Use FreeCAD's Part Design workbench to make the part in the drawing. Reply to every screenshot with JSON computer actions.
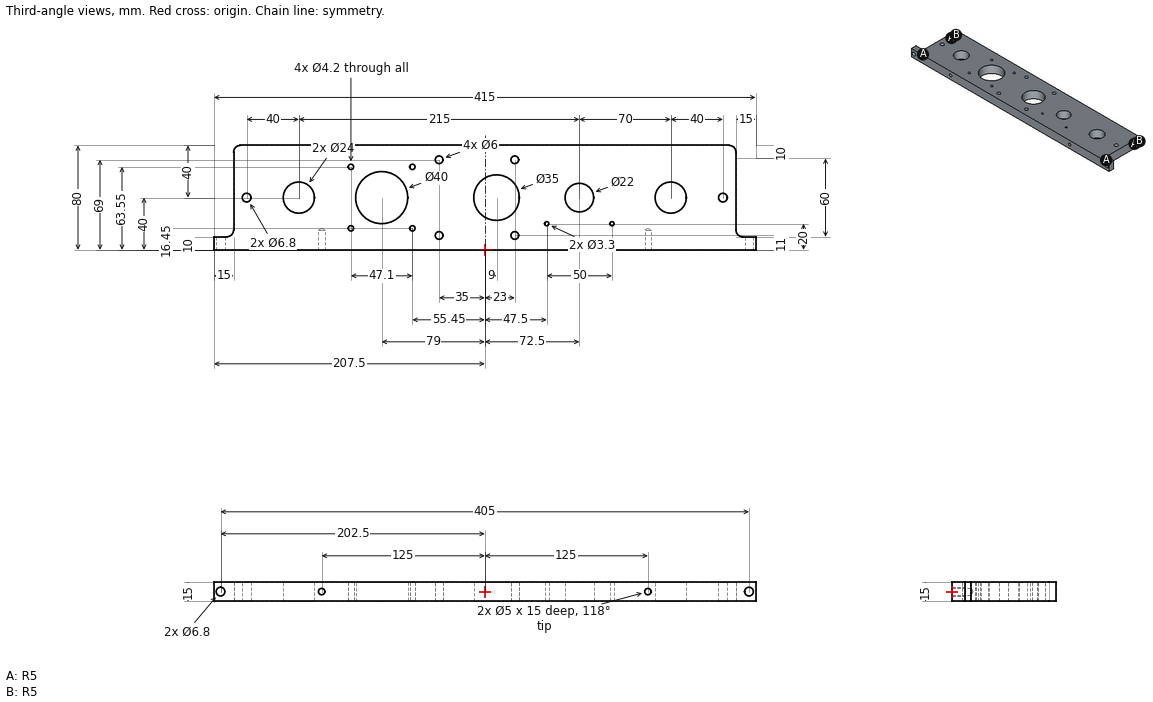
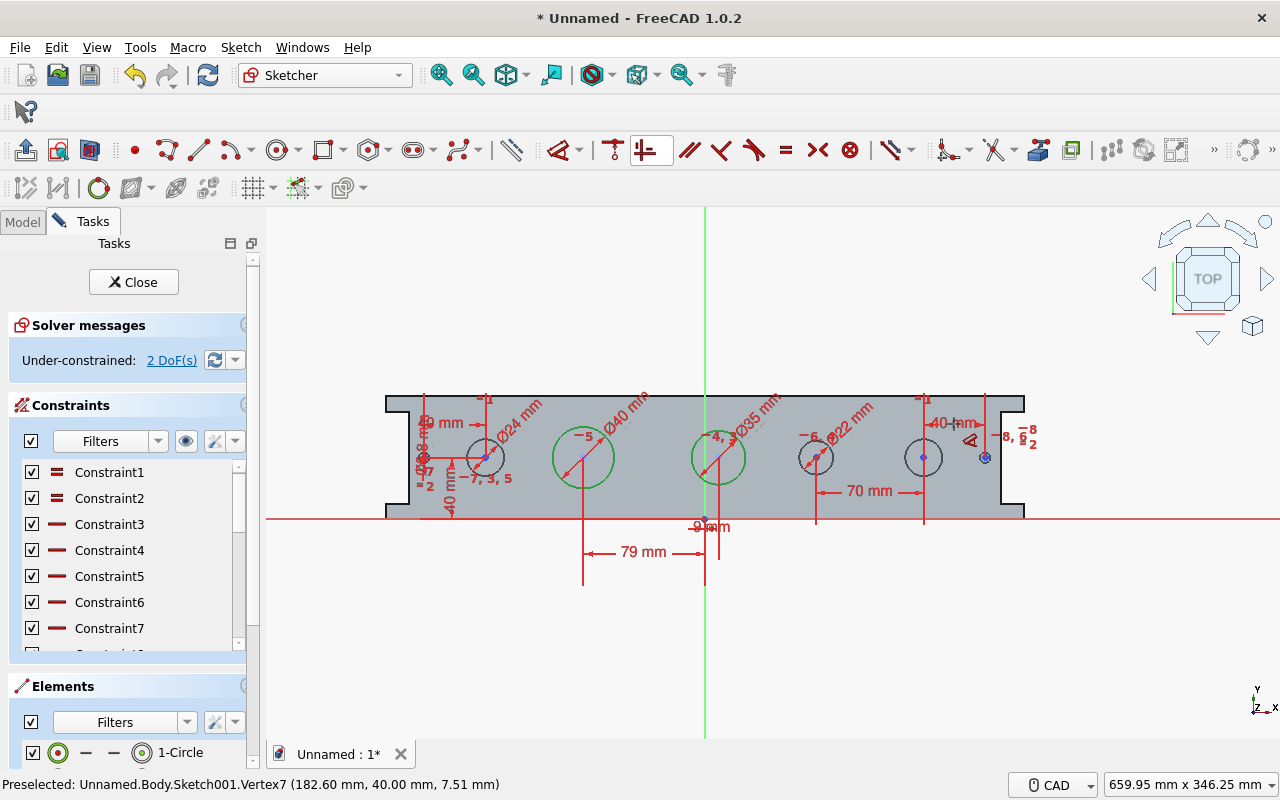
{"action": "left_click", "coordinate": [816, 458]}
{"action": "left_click", "coordinate": [760, 553]}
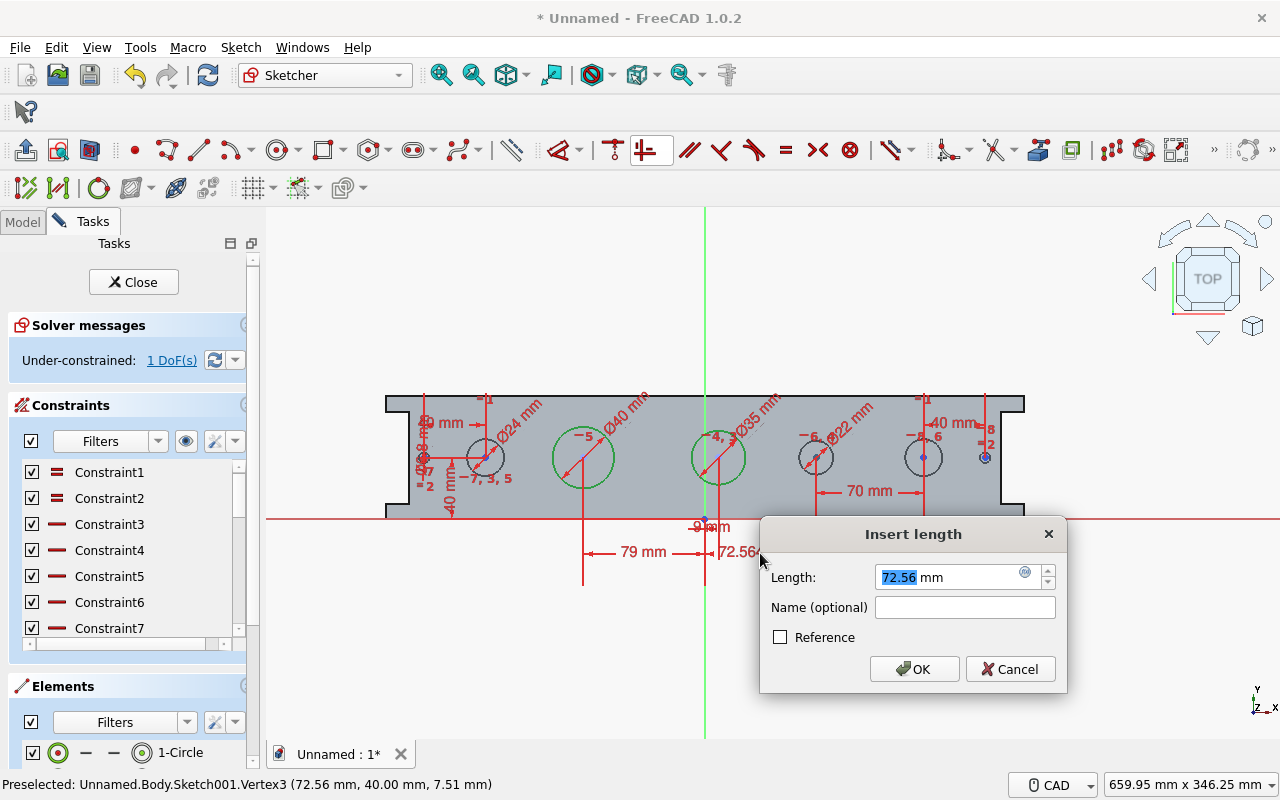
{"action": "type", "text": "72.5"}
{"action": "key", "text": "Return"}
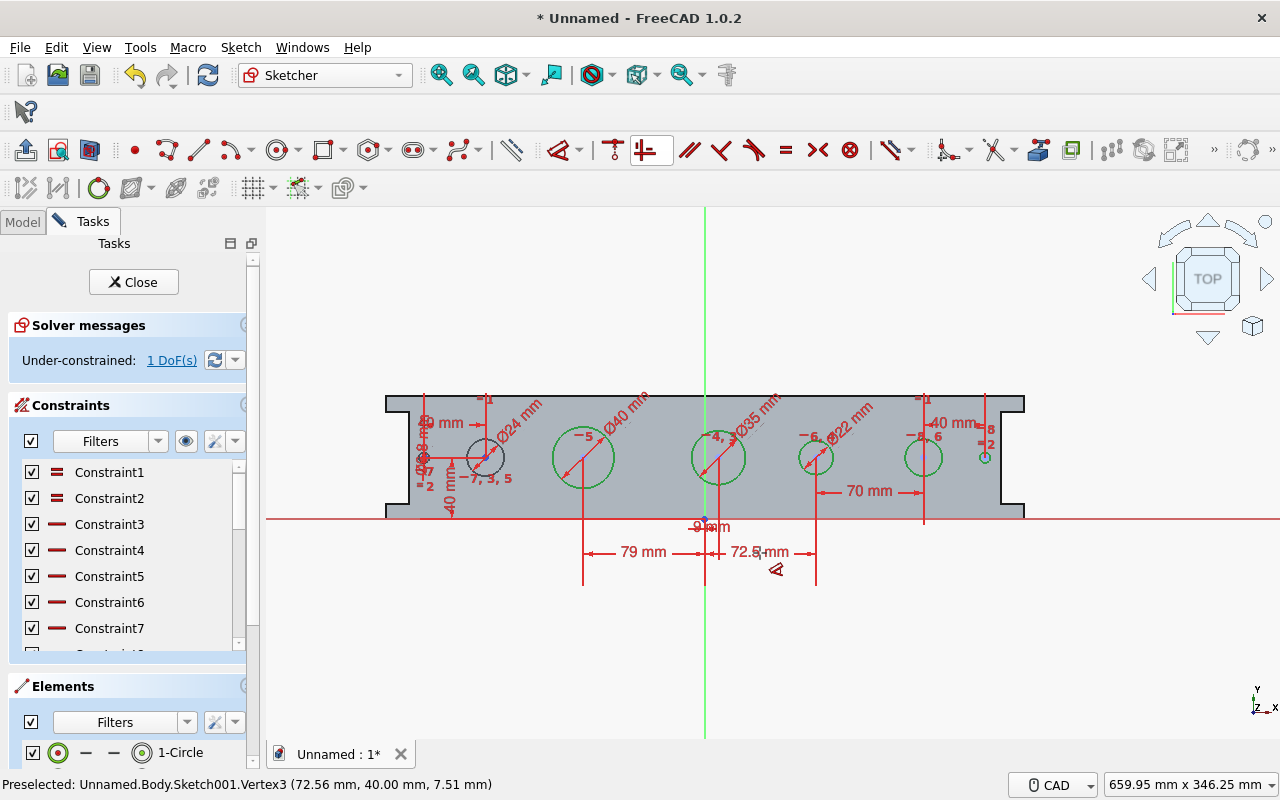
{"action": "left_click", "coordinate": [486, 458]}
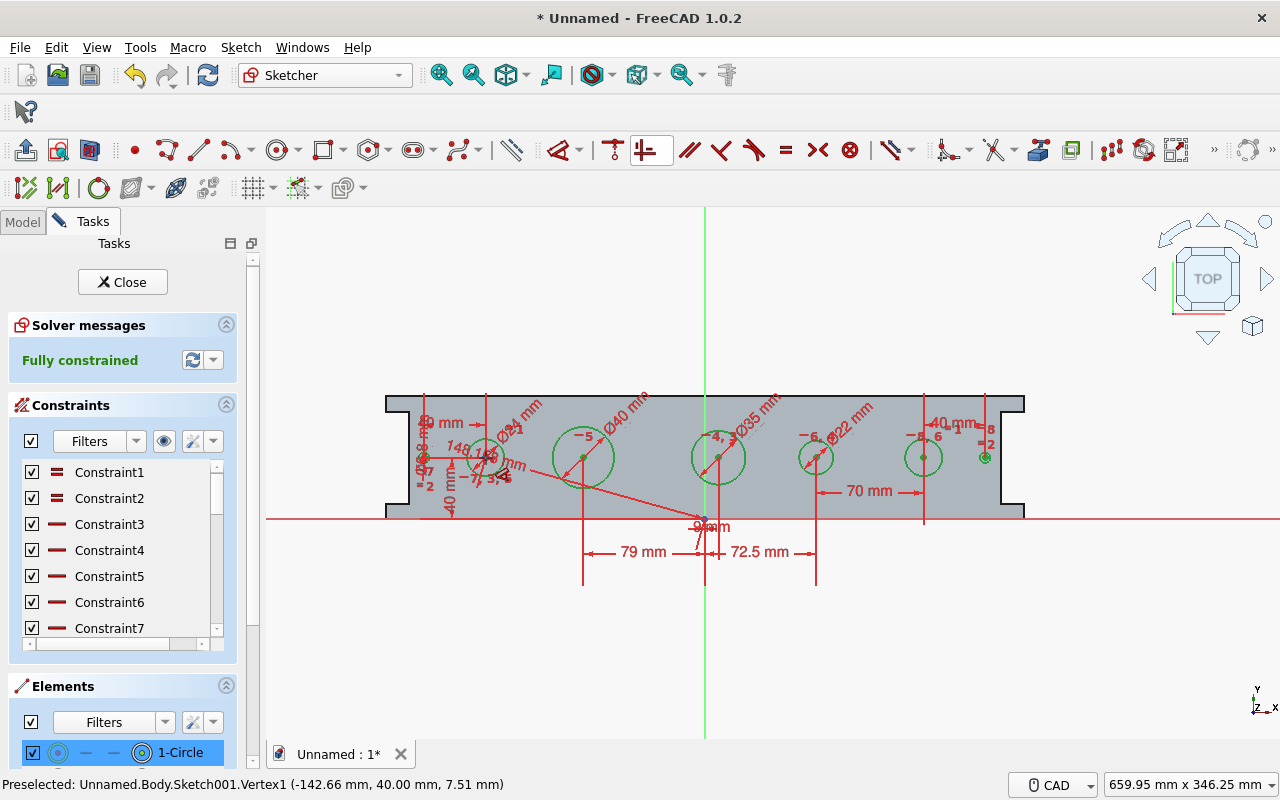
{"action": "left_click", "coordinate": [816, 458]}
{"action": "left_click", "coordinate": [651, 492]}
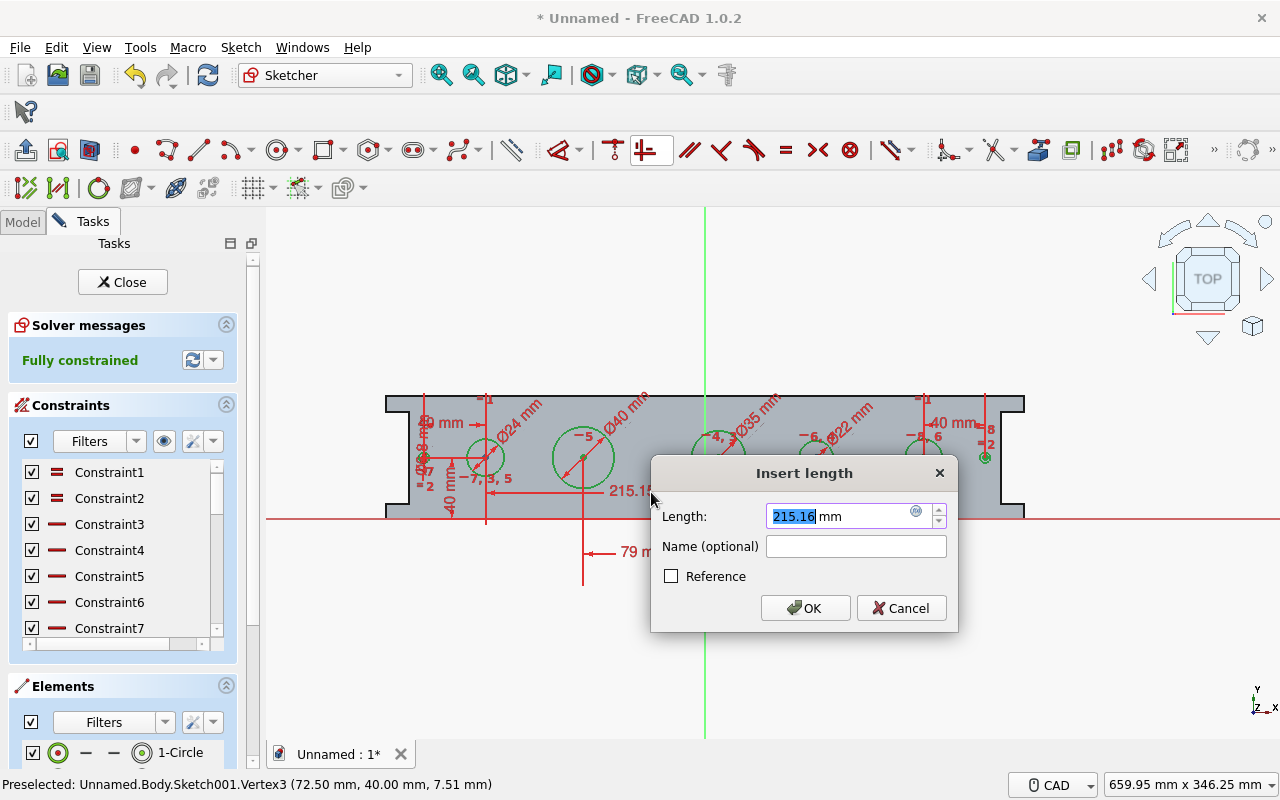
{"action": "type", "text": "215"}
{"action": "key", "text": "Return"}
{"action": "key", "text": "Escape"}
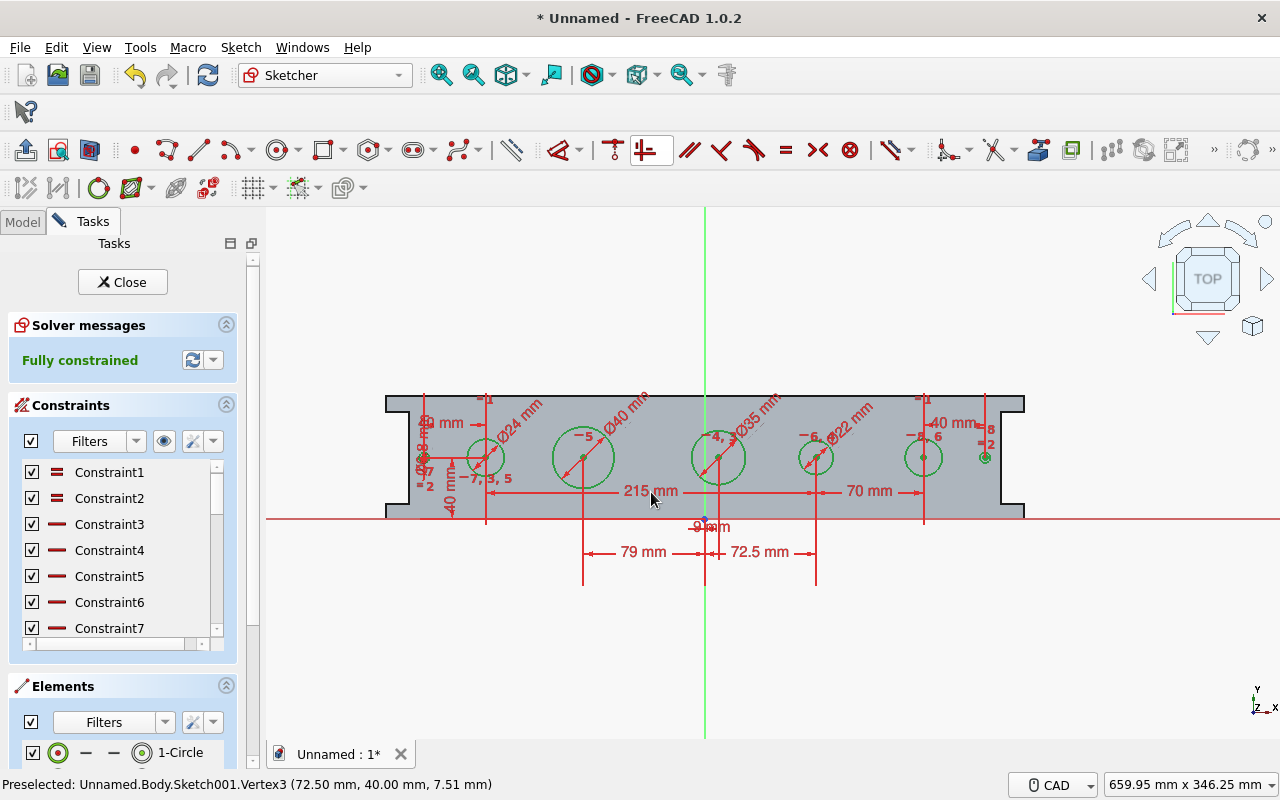
{"action": "left_click", "coordinate": [123, 282]}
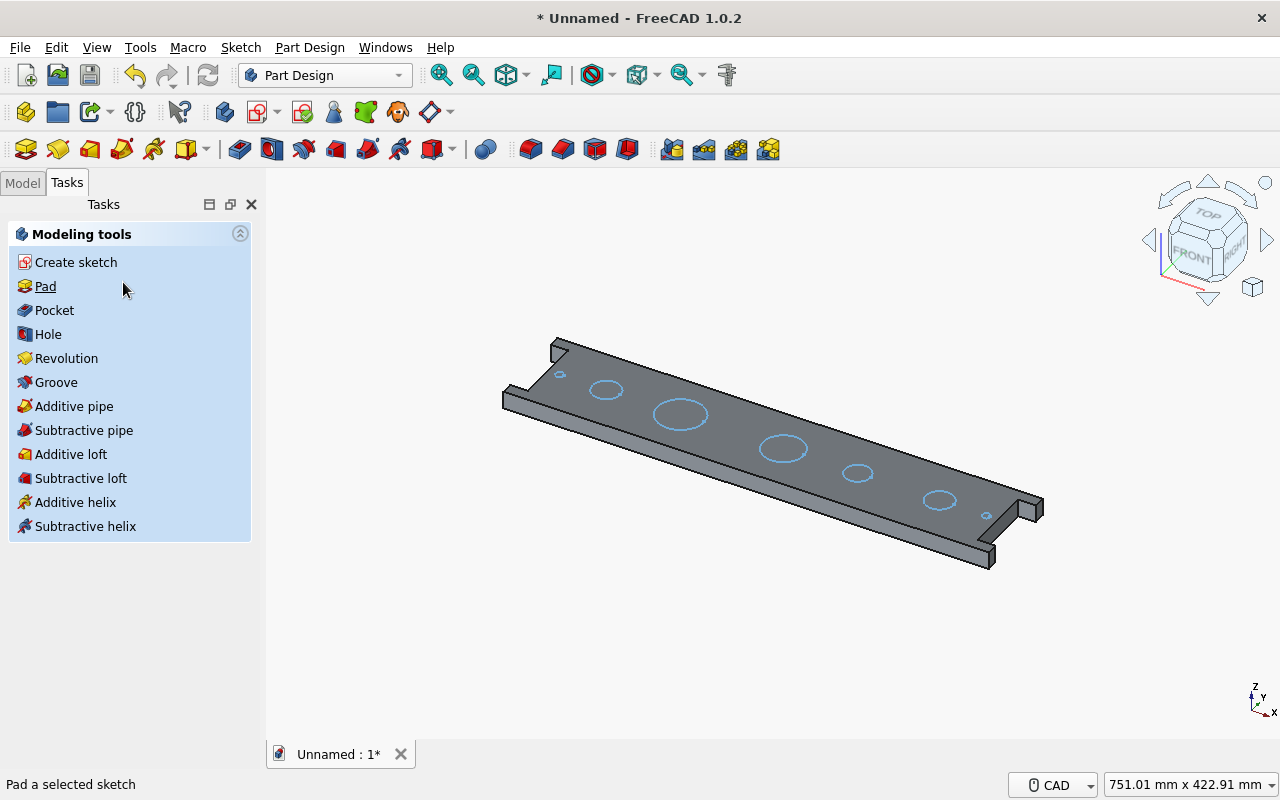
{"action": "left_click", "coordinate": [240, 150]}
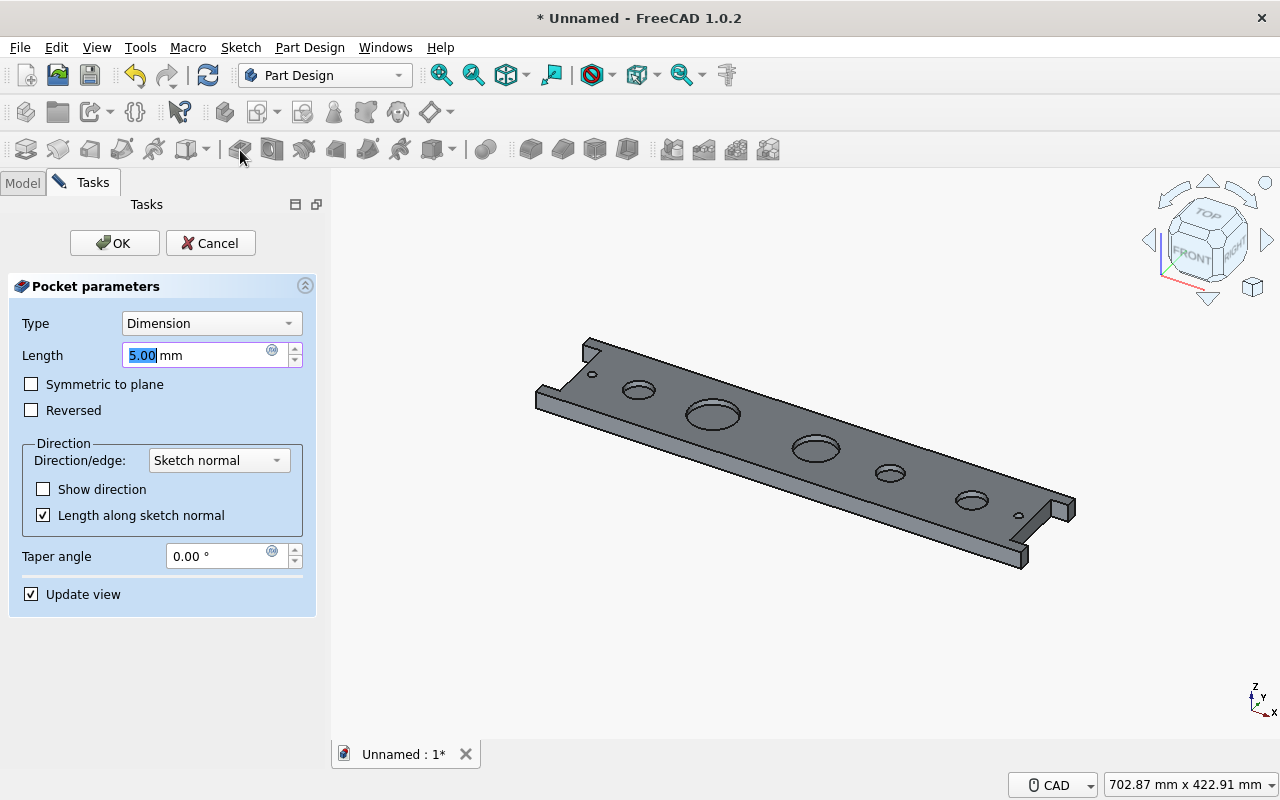
{"action": "type", "text": "15"}
{"action": "key", "text": "Tab"}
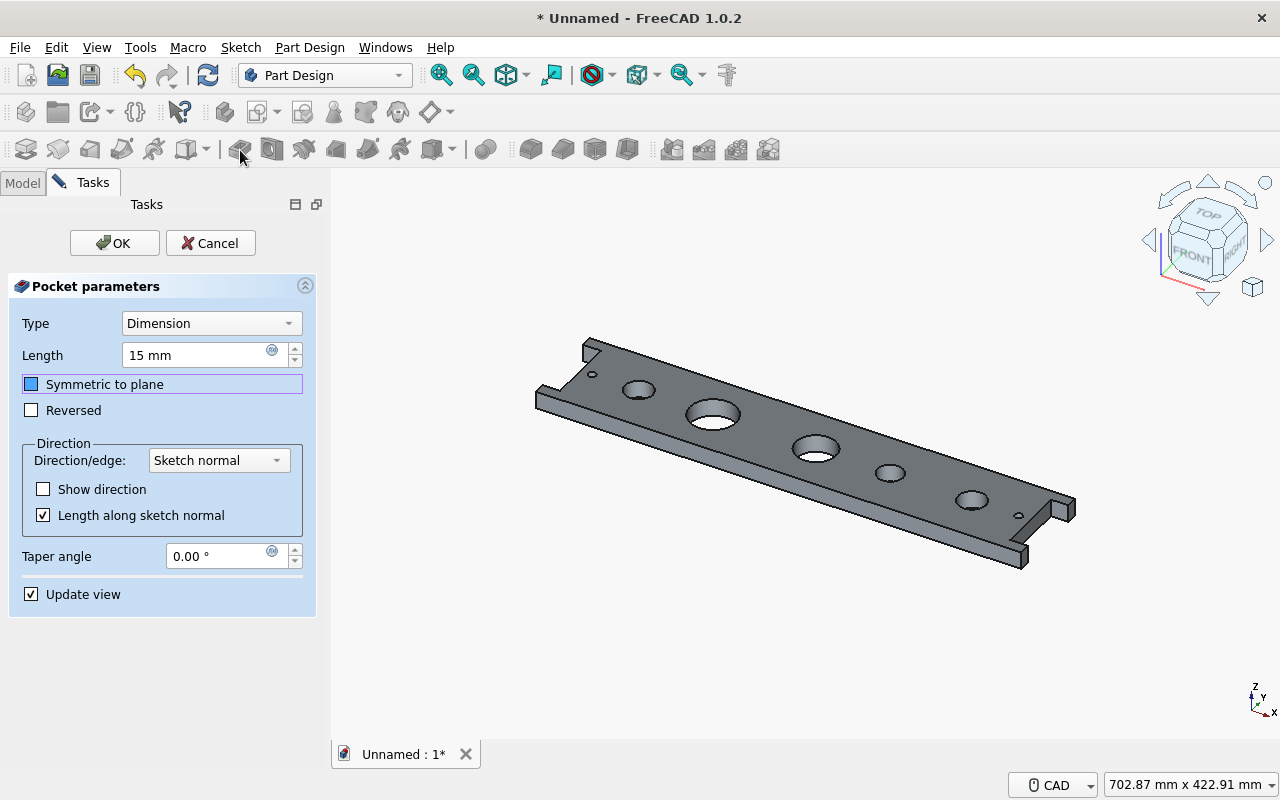
{"action": "left_click", "coordinate": [115, 243]}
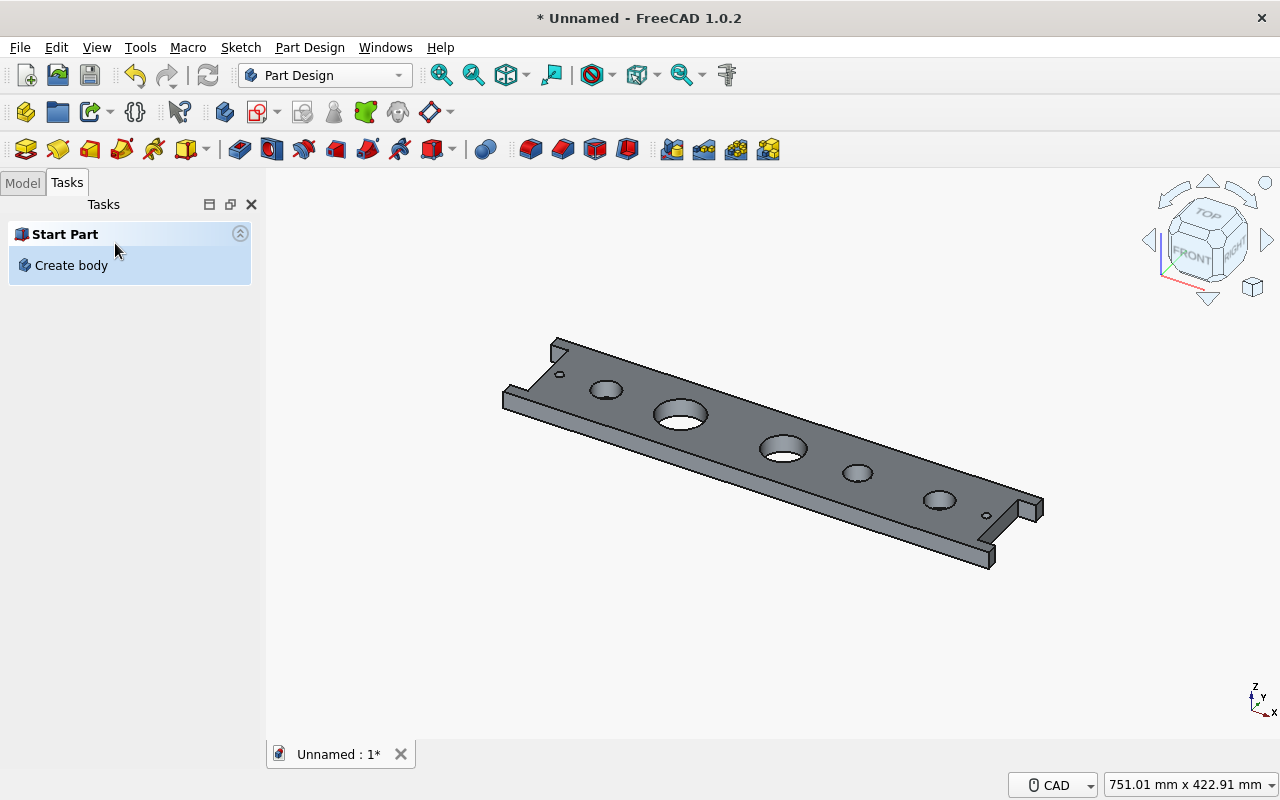
{"action": "left_click", "coordinate": [927, 475]}